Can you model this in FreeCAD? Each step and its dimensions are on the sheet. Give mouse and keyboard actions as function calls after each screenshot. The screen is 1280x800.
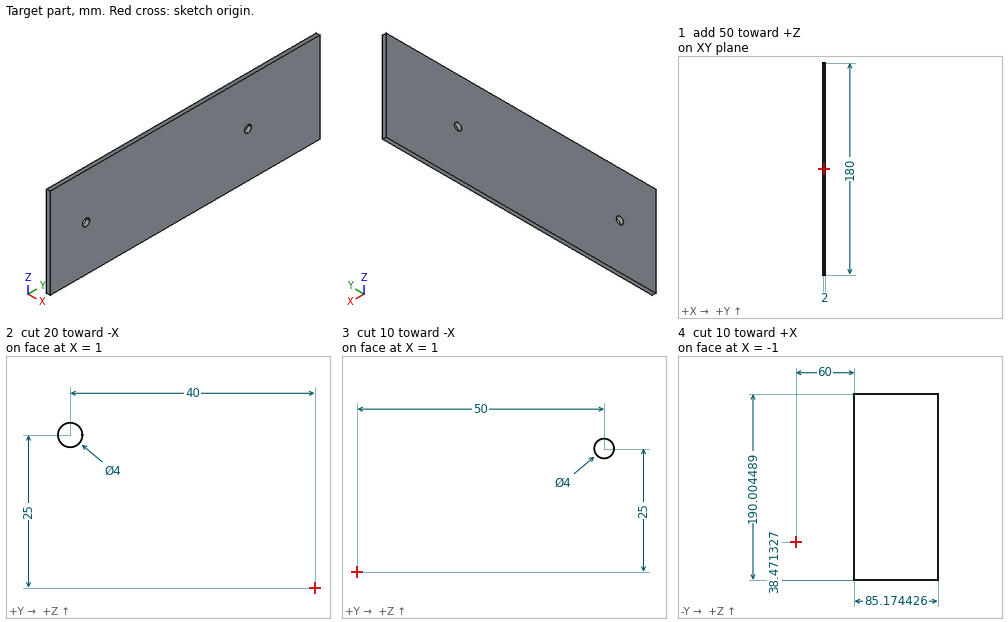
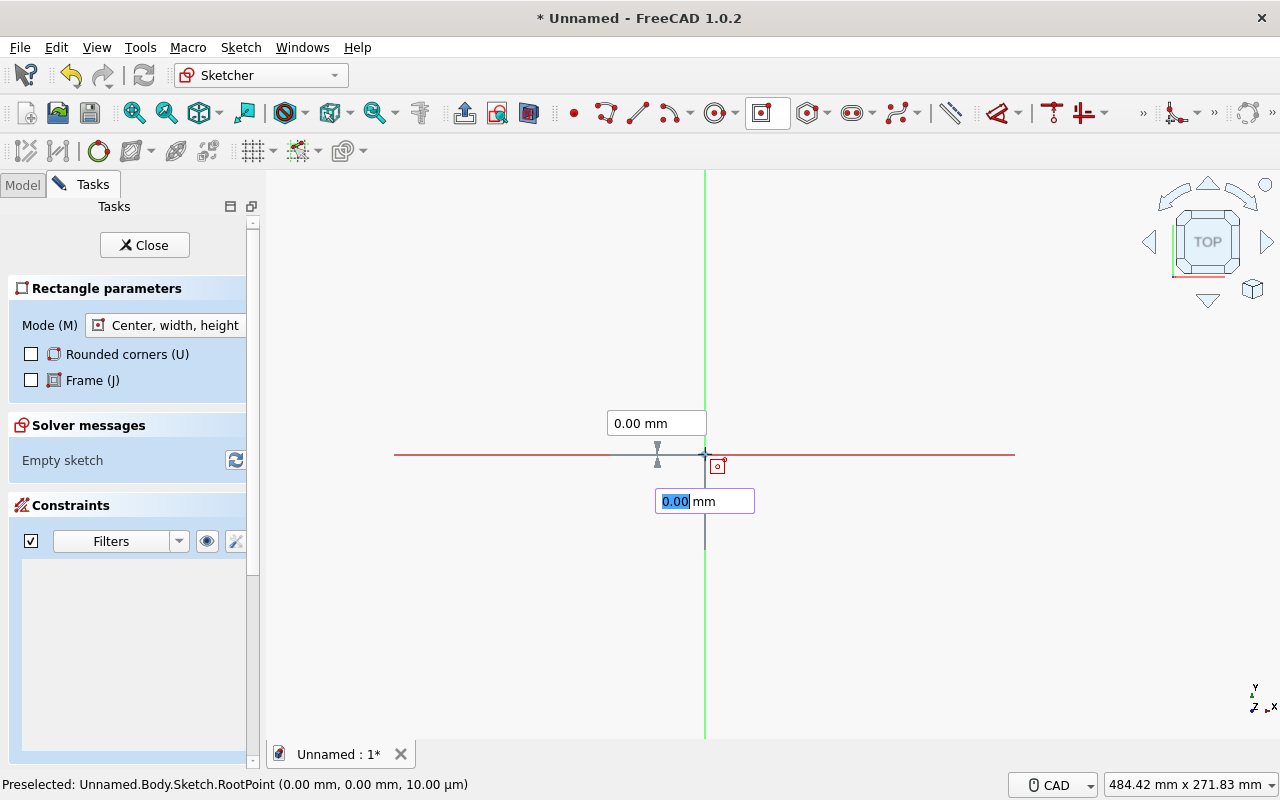
scroll(707, 266, up, 11)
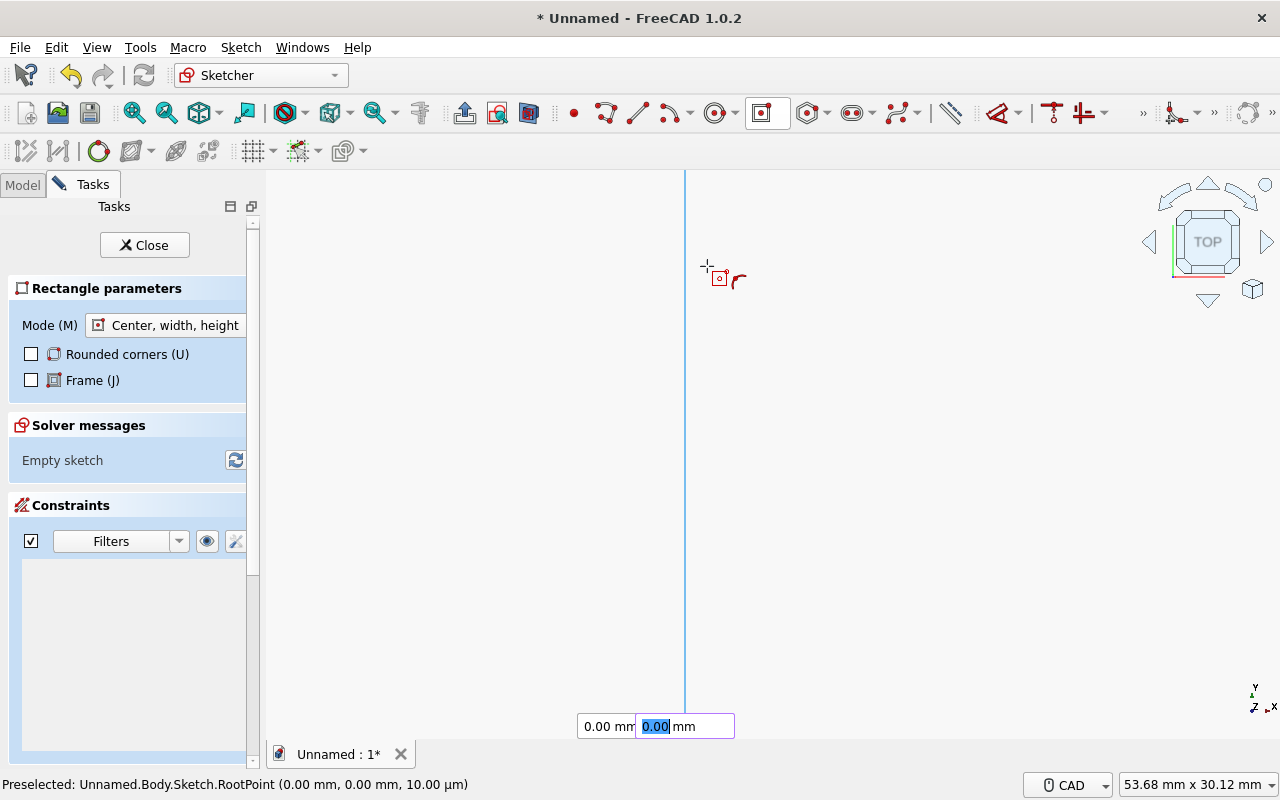
click(704, 266)
key(Escape)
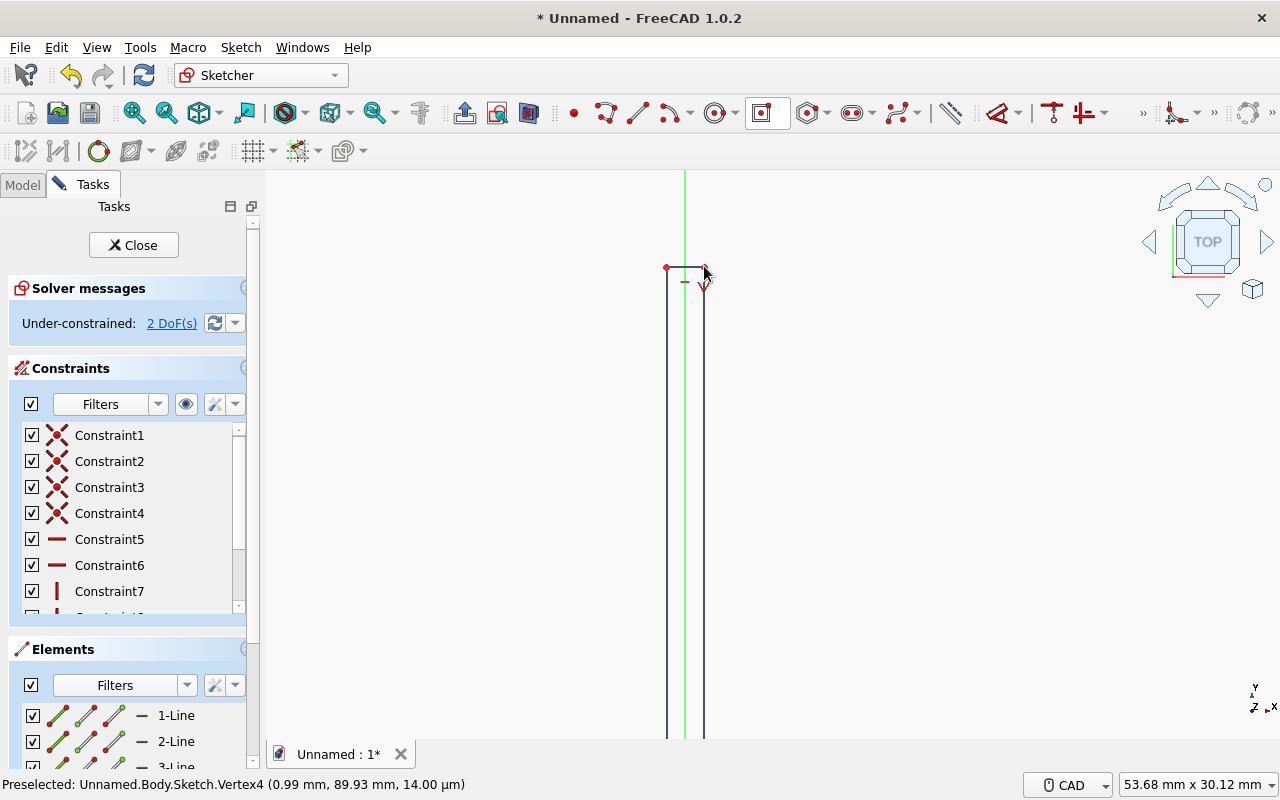
scroll(707, 266, down, 11)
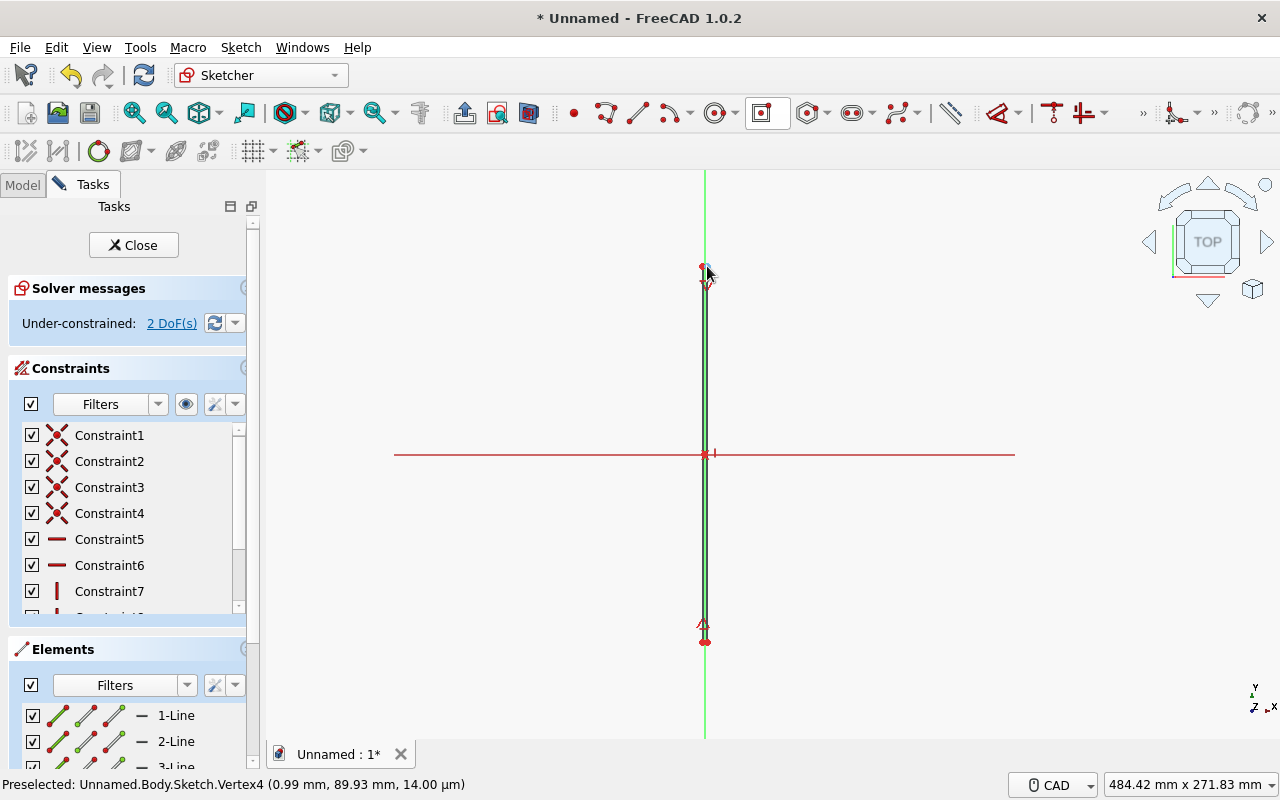
scroll(705, 643, up, 12)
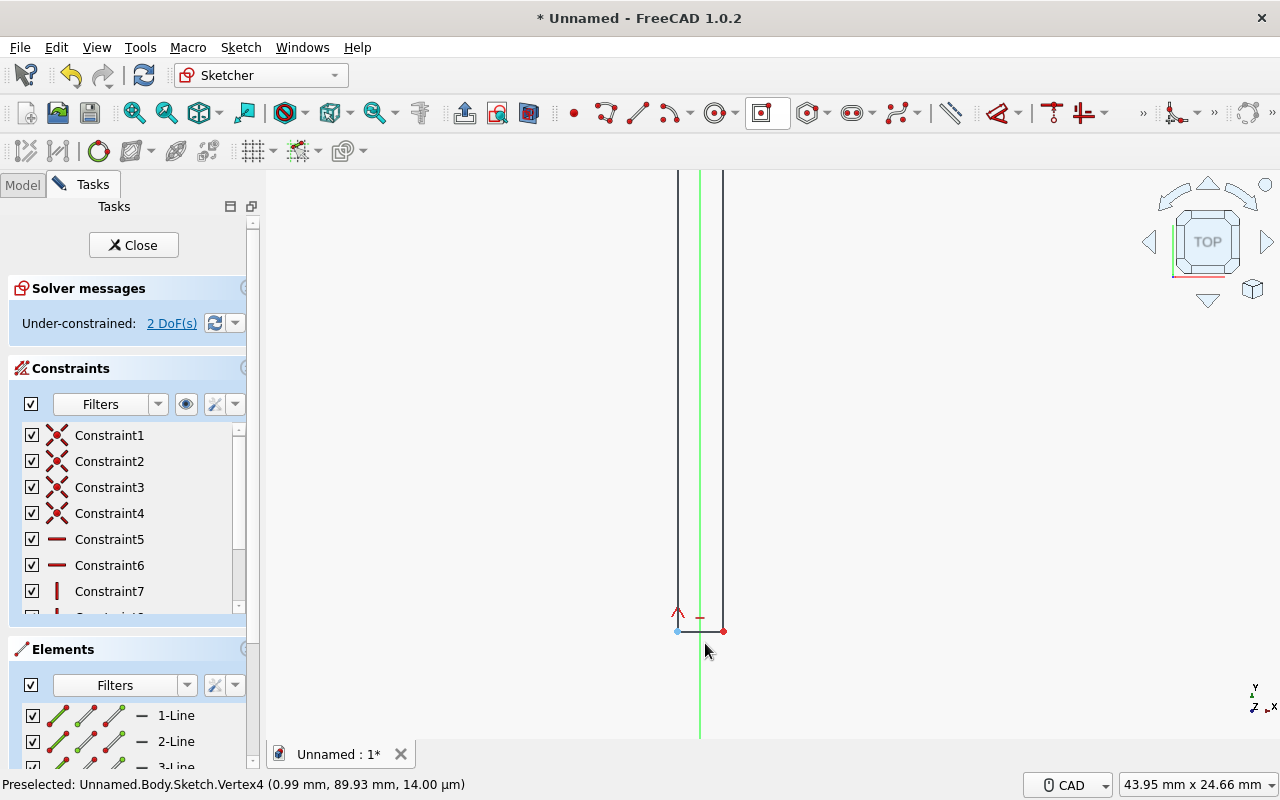
click(696, 632)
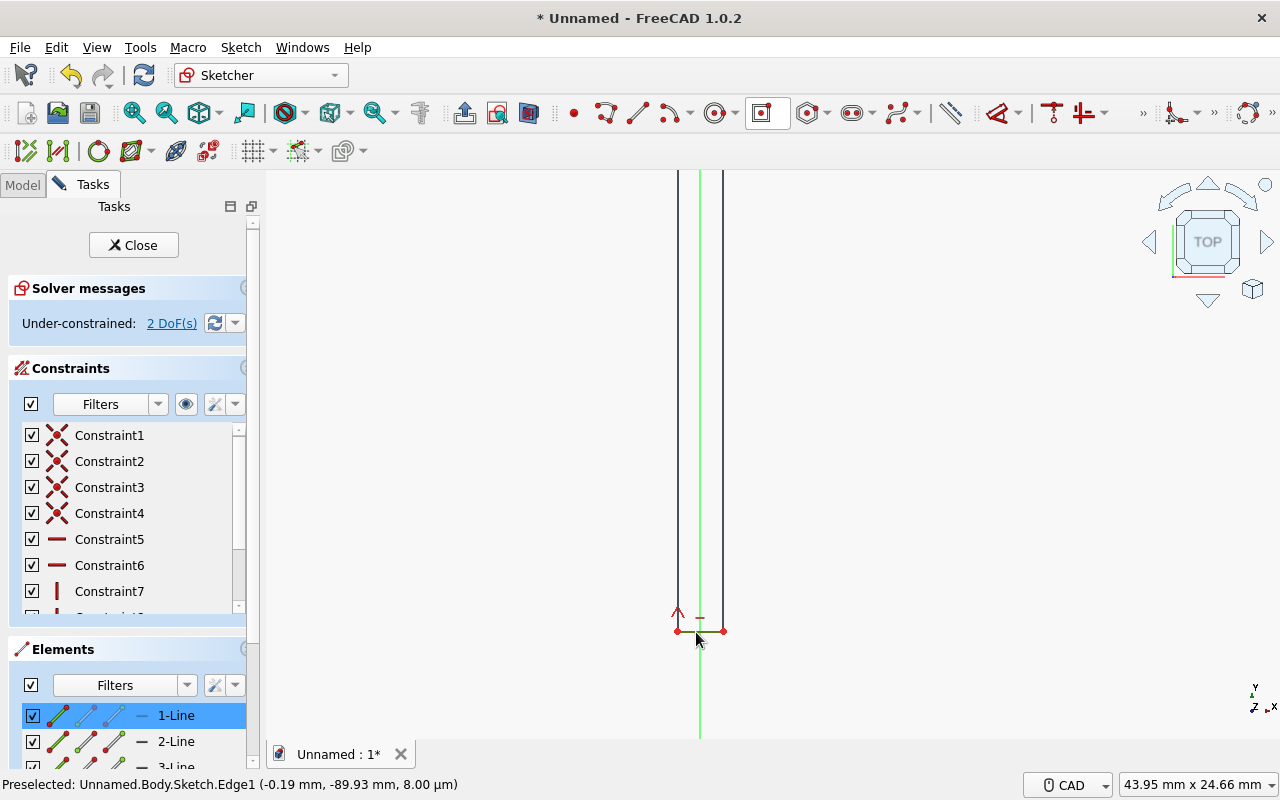
click(1020, 114)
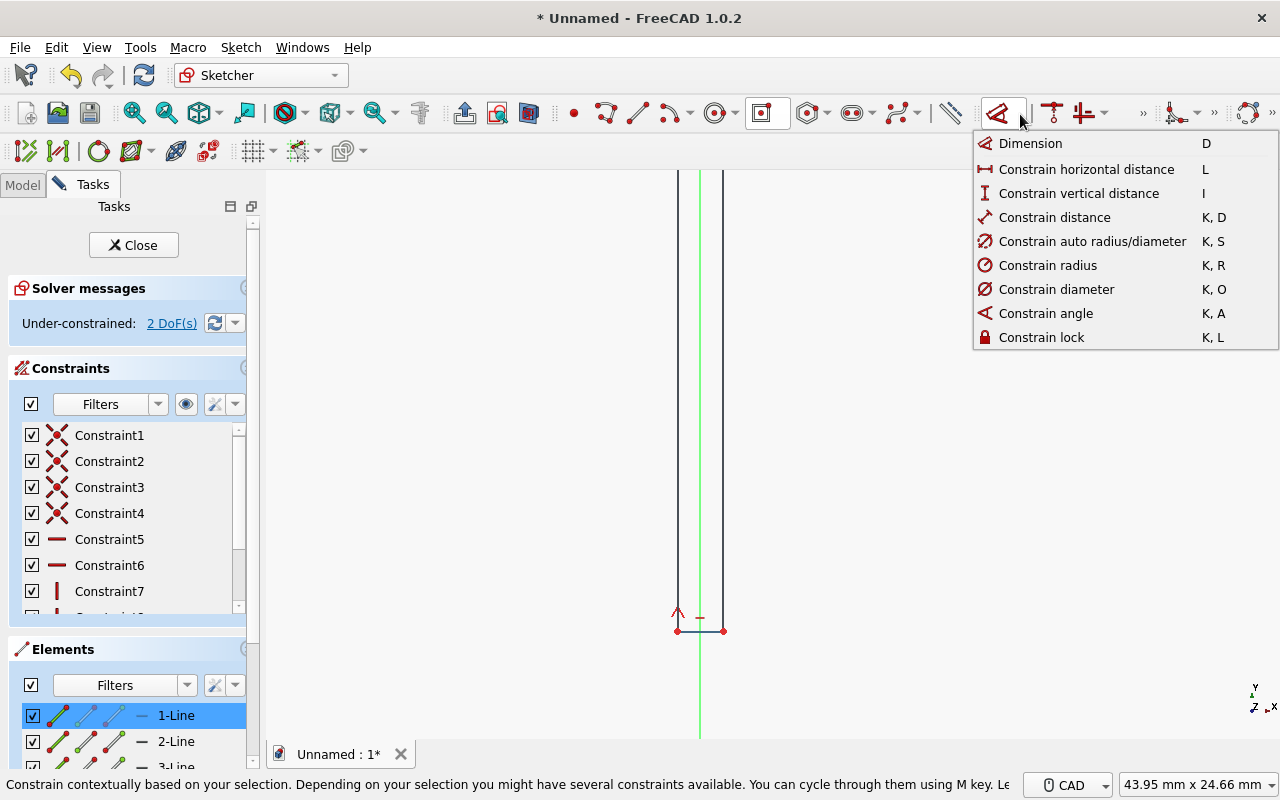
click(1126, 169)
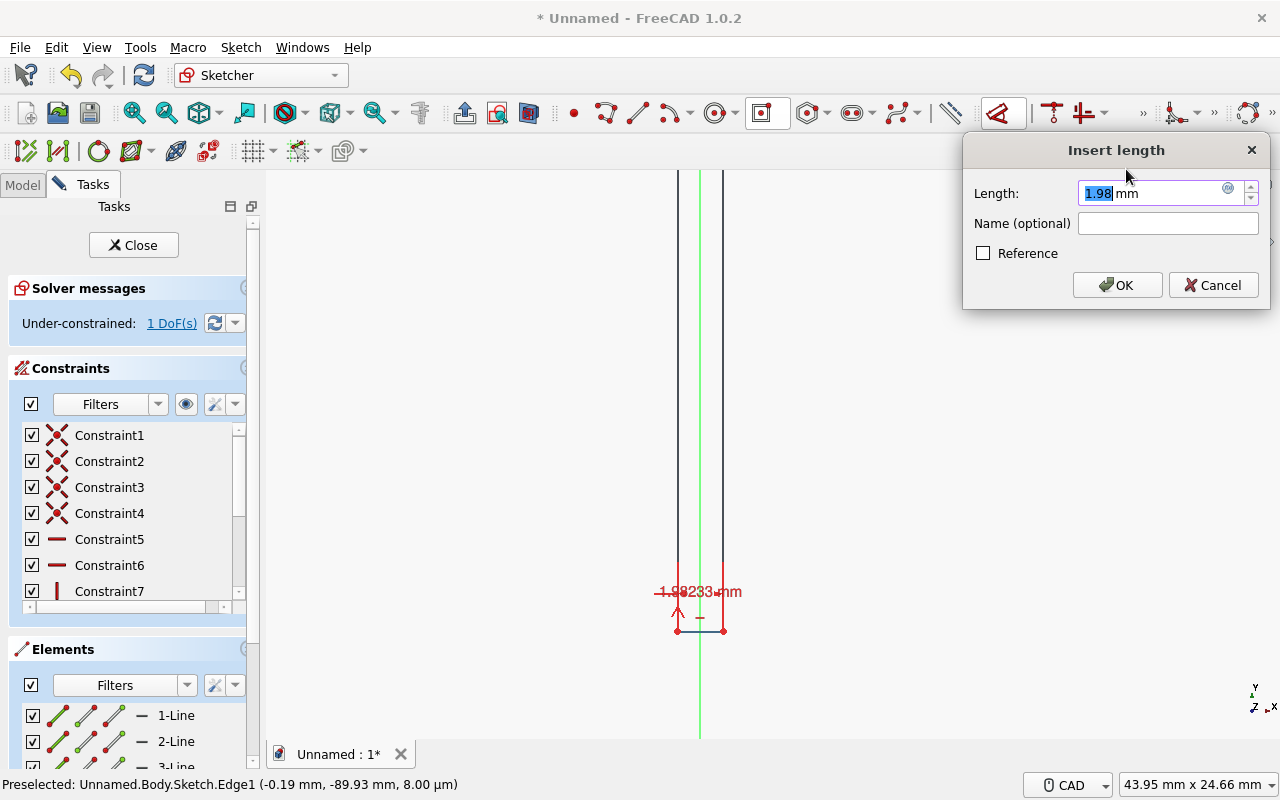
text(2)
key(Return)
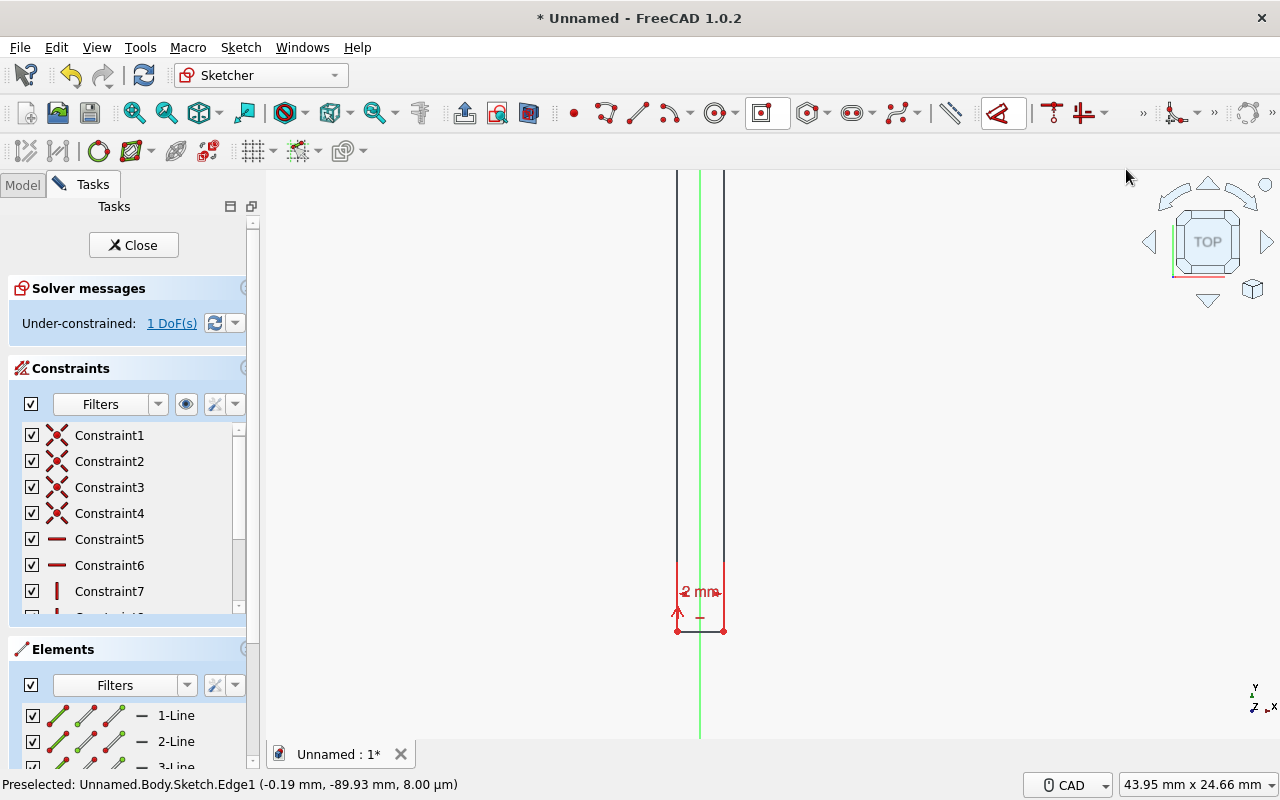
scroll(705, 644, down, 12)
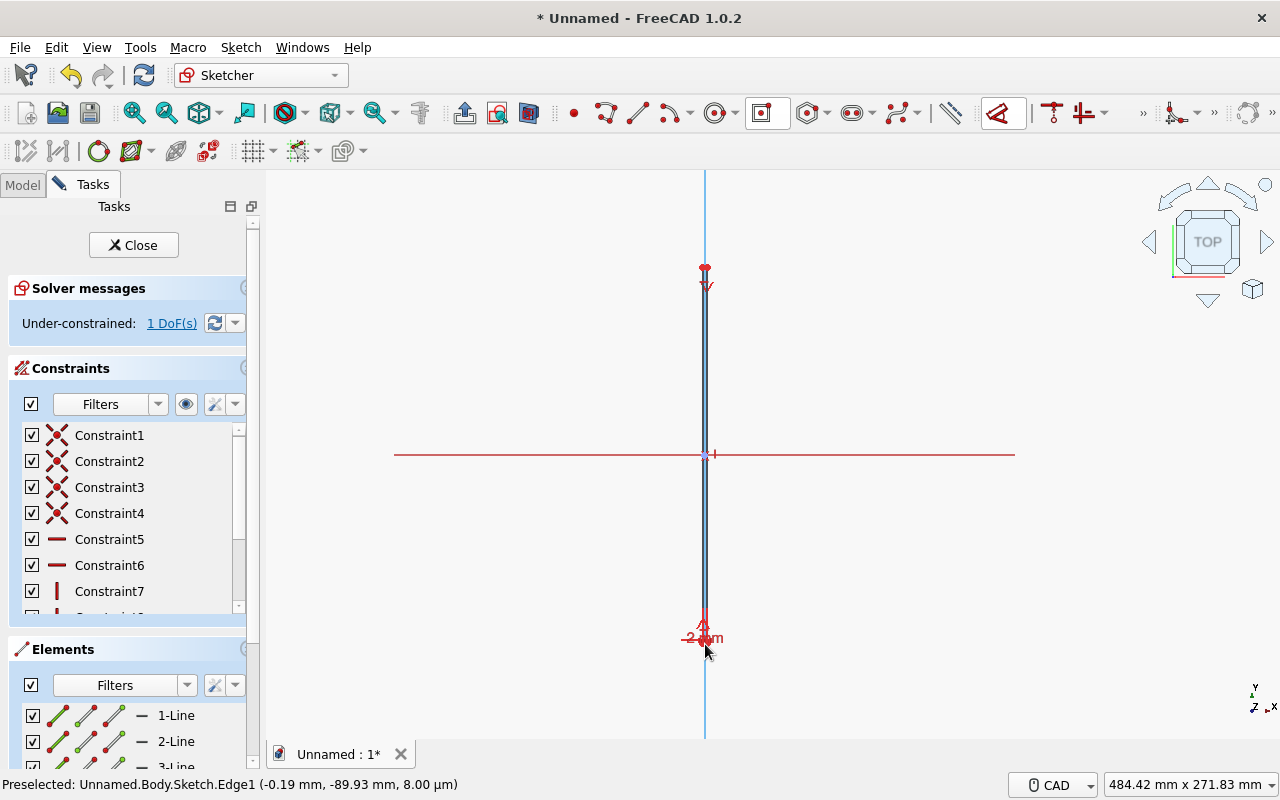
scroll(707, 531, up, 10)